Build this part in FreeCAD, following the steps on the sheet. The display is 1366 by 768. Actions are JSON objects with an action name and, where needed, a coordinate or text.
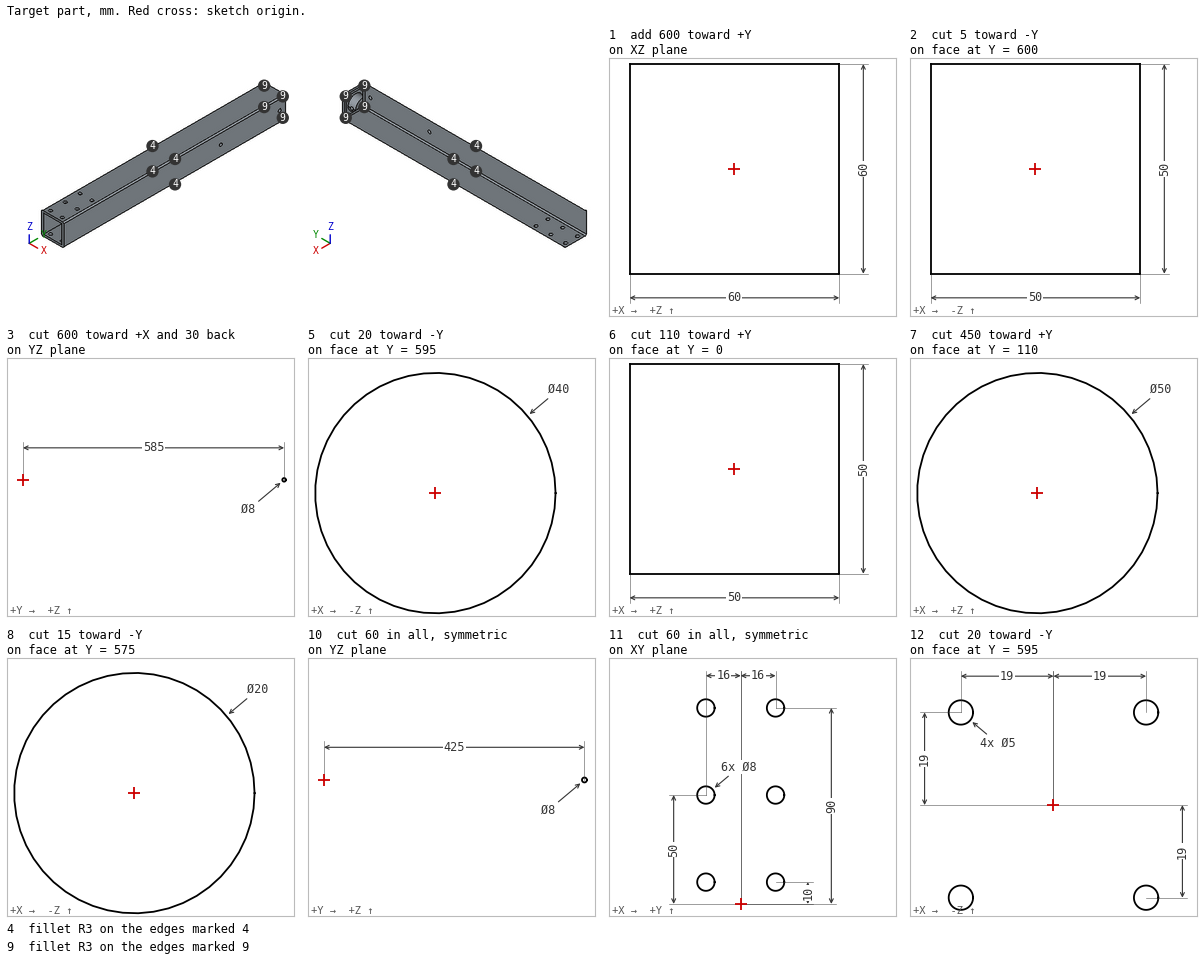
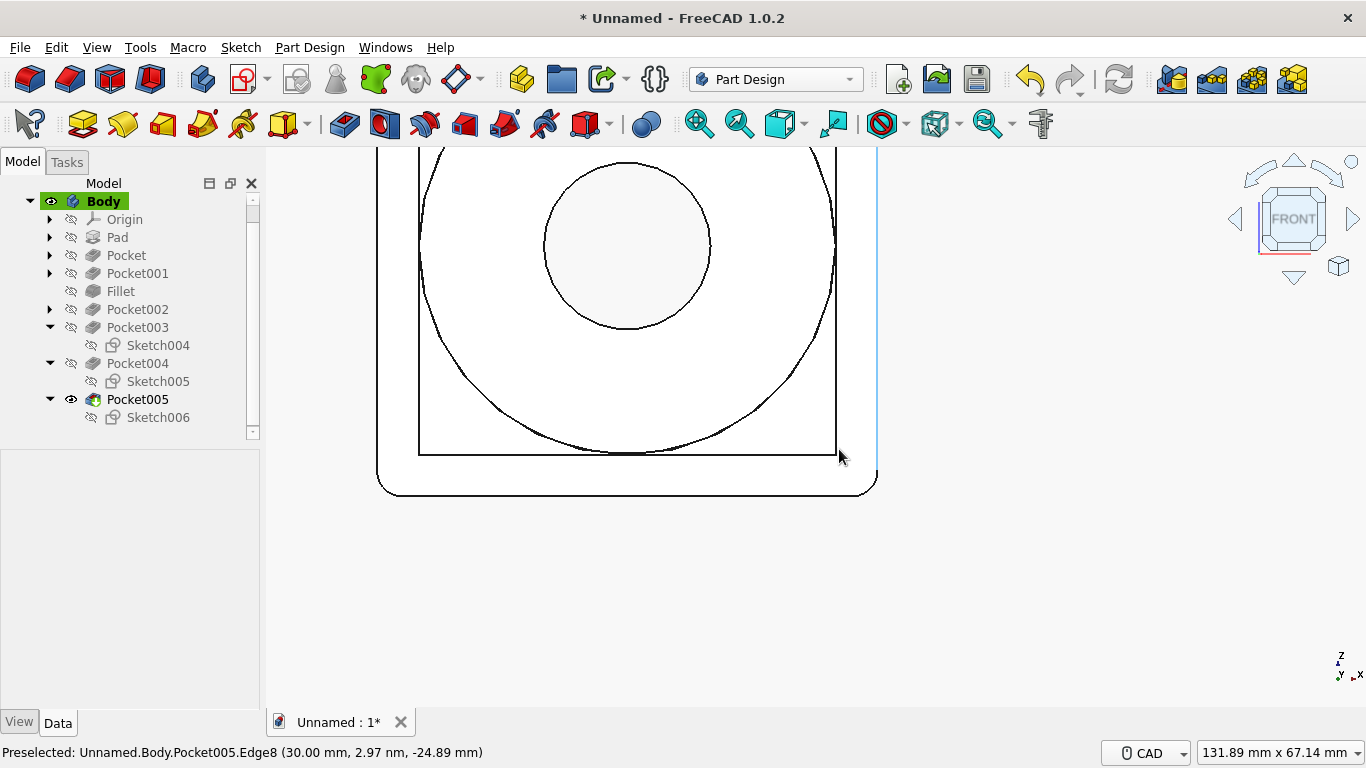
{"action": "left_click", "coordinate": [700, 124]}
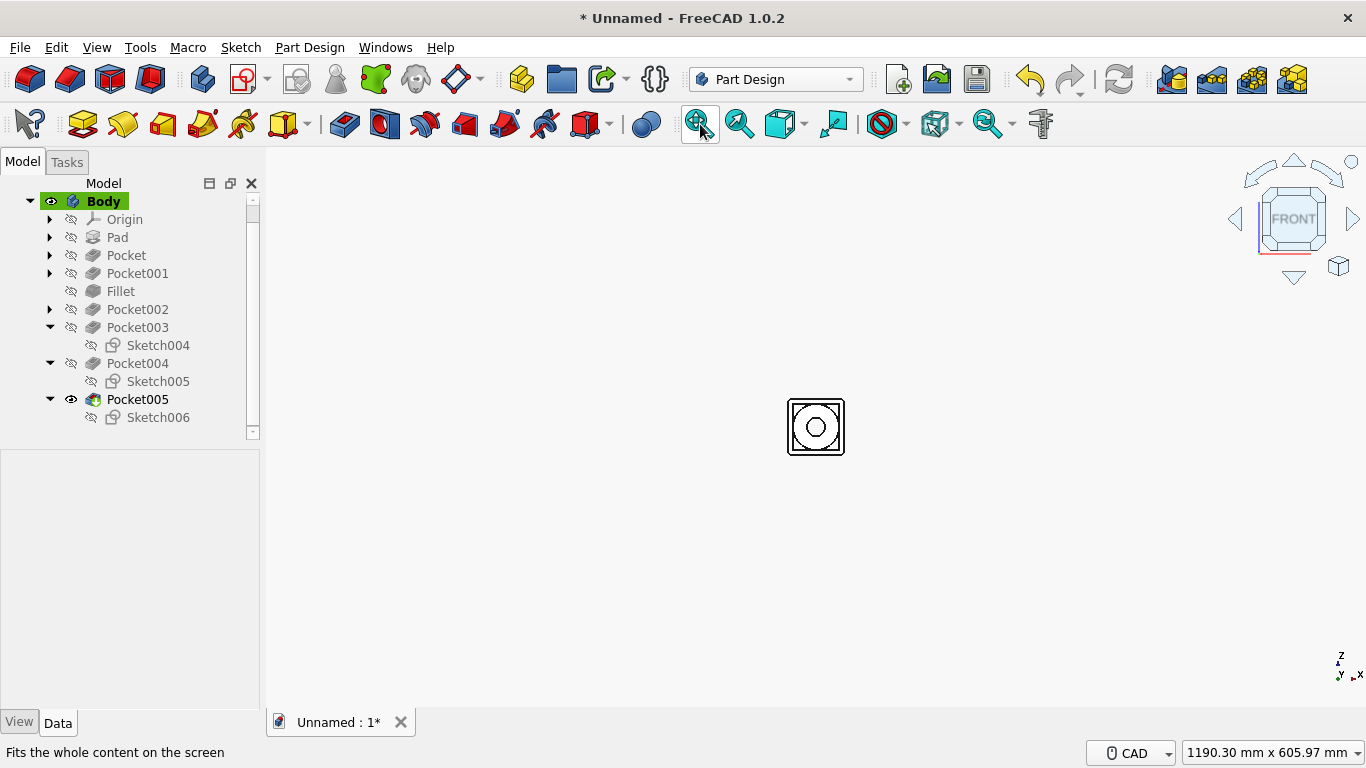
{"action": "key", "text": "3"}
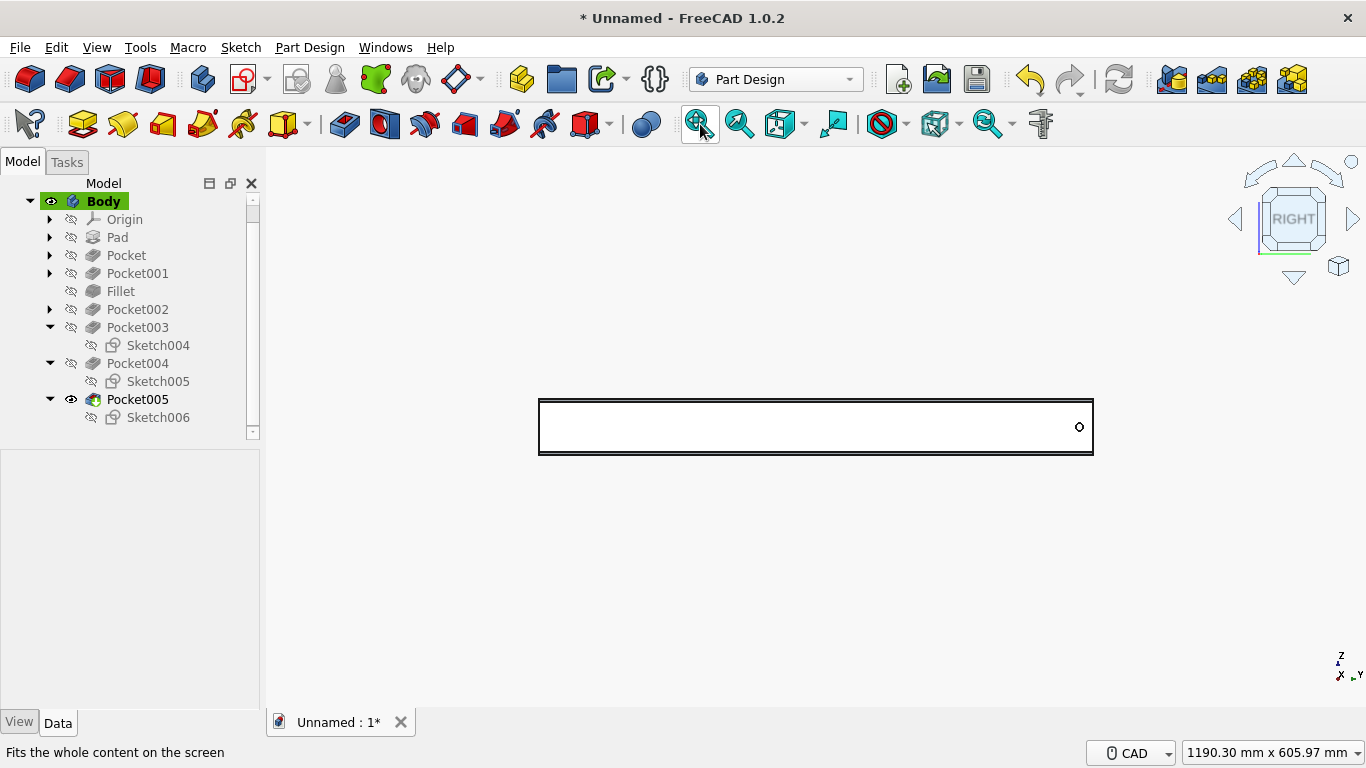
{"action": "scroll", "coordinate": [1091, 449], "scroll_direction": "up", "scroll_amount": 11}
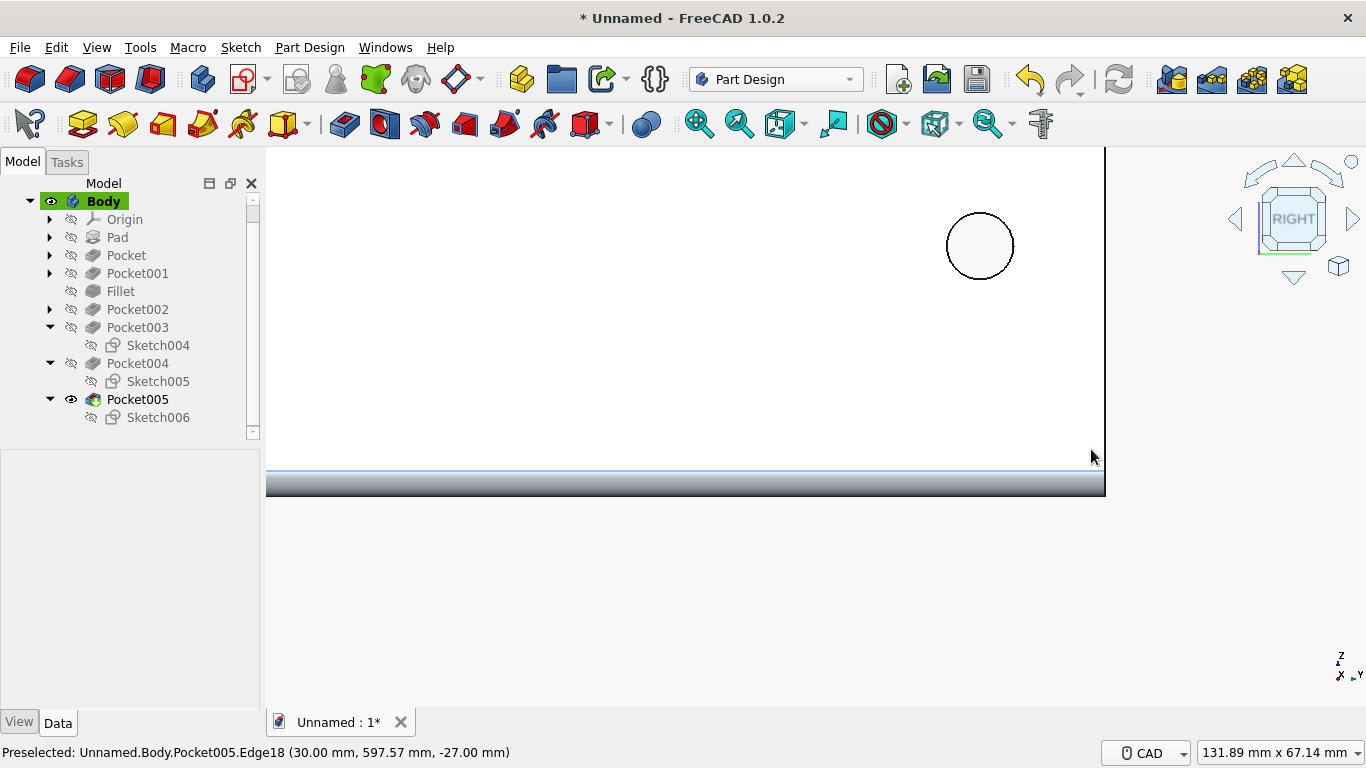
{"action": "left_click", "coordinate": [700, 124]}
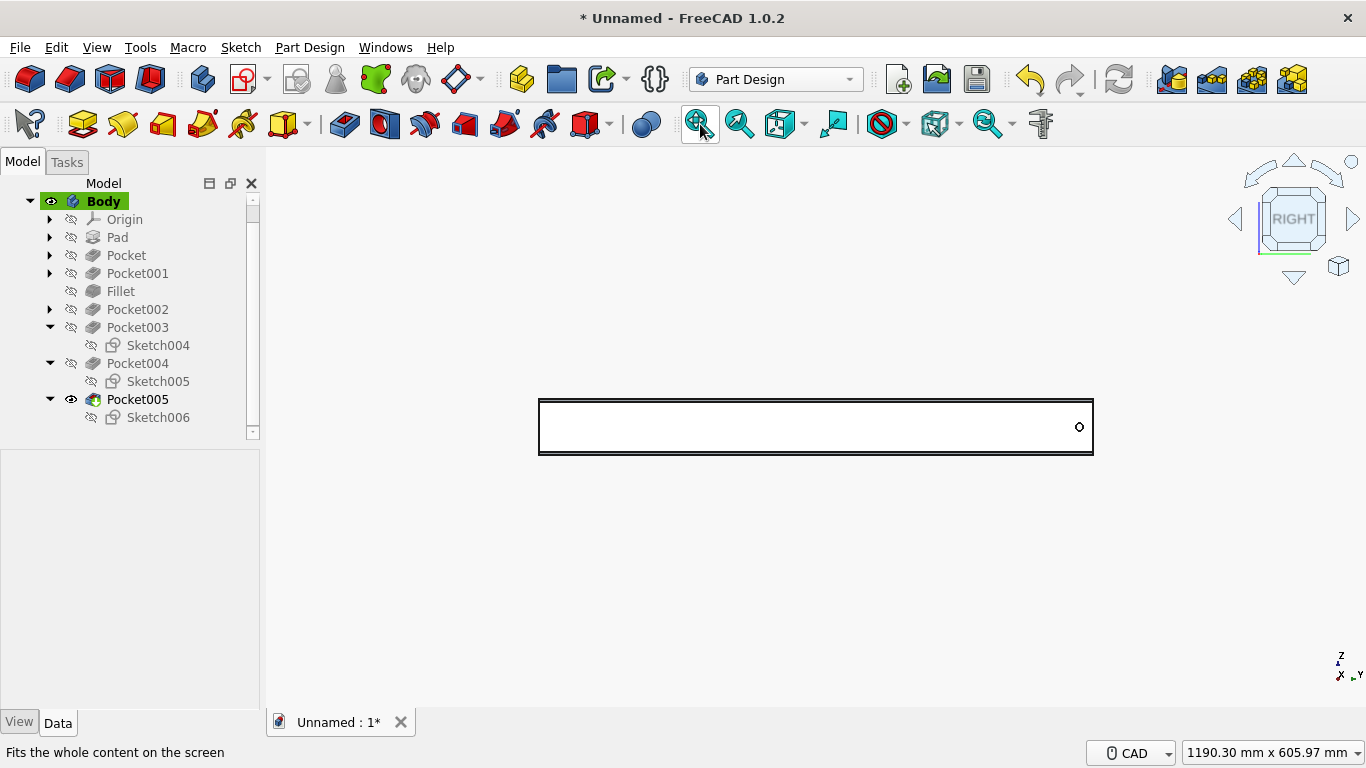
{"action": "key", "text": "5"}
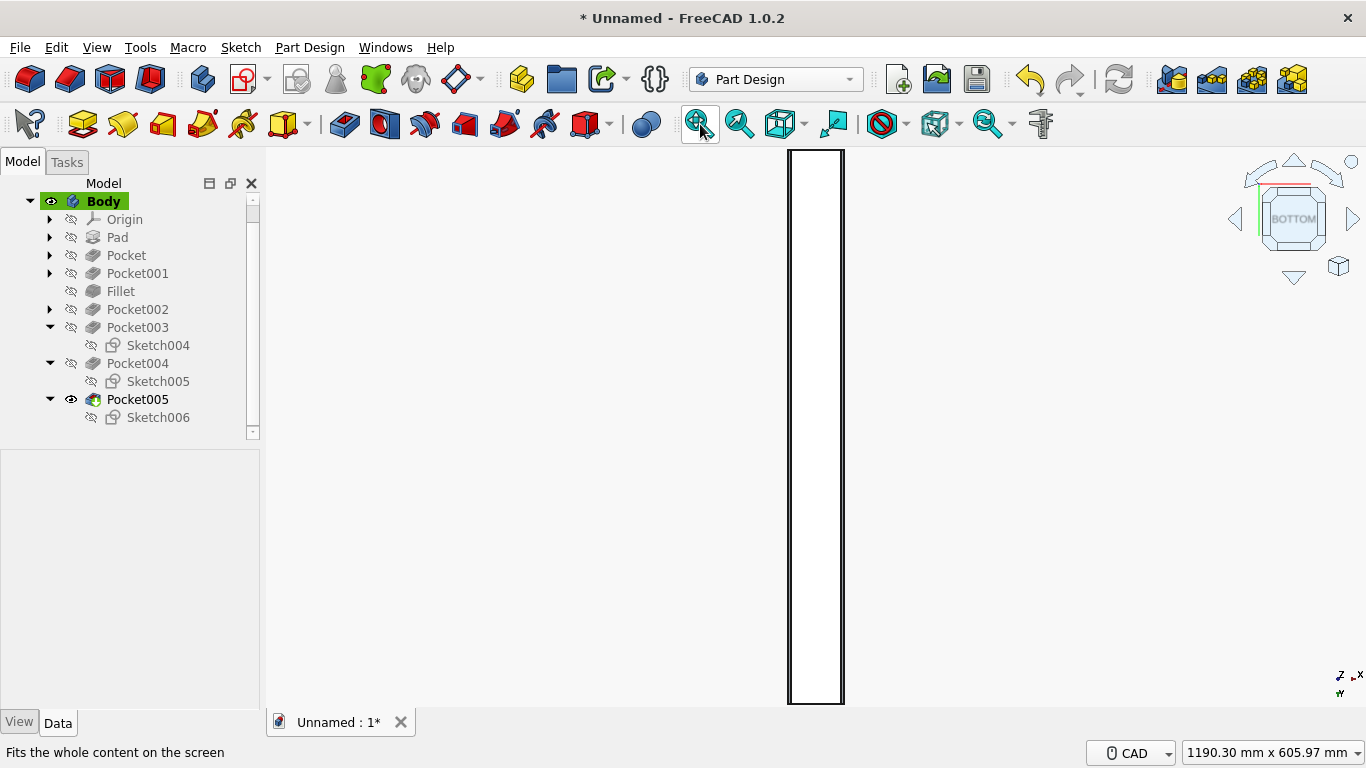
{"action": "key", "text": "4"}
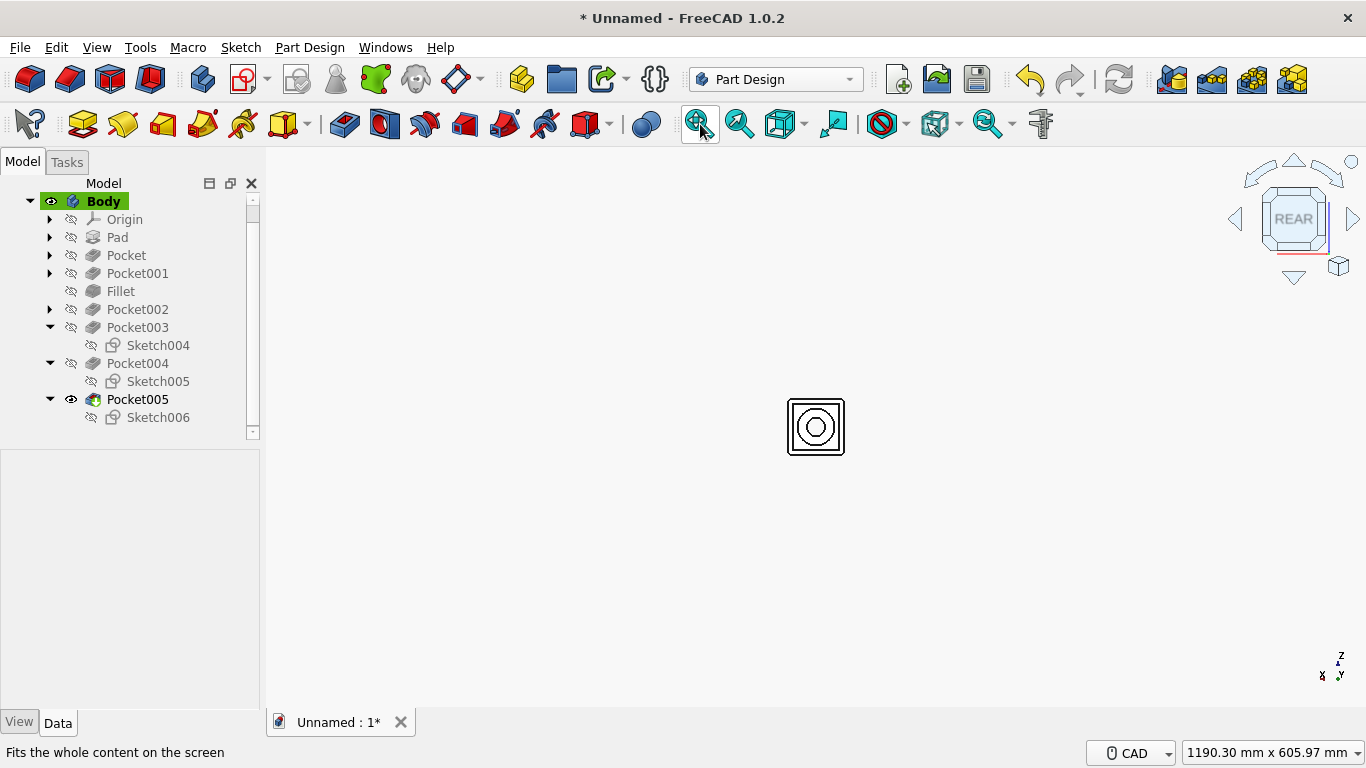
{"action": "left_click", "coordinate": [700, 124]}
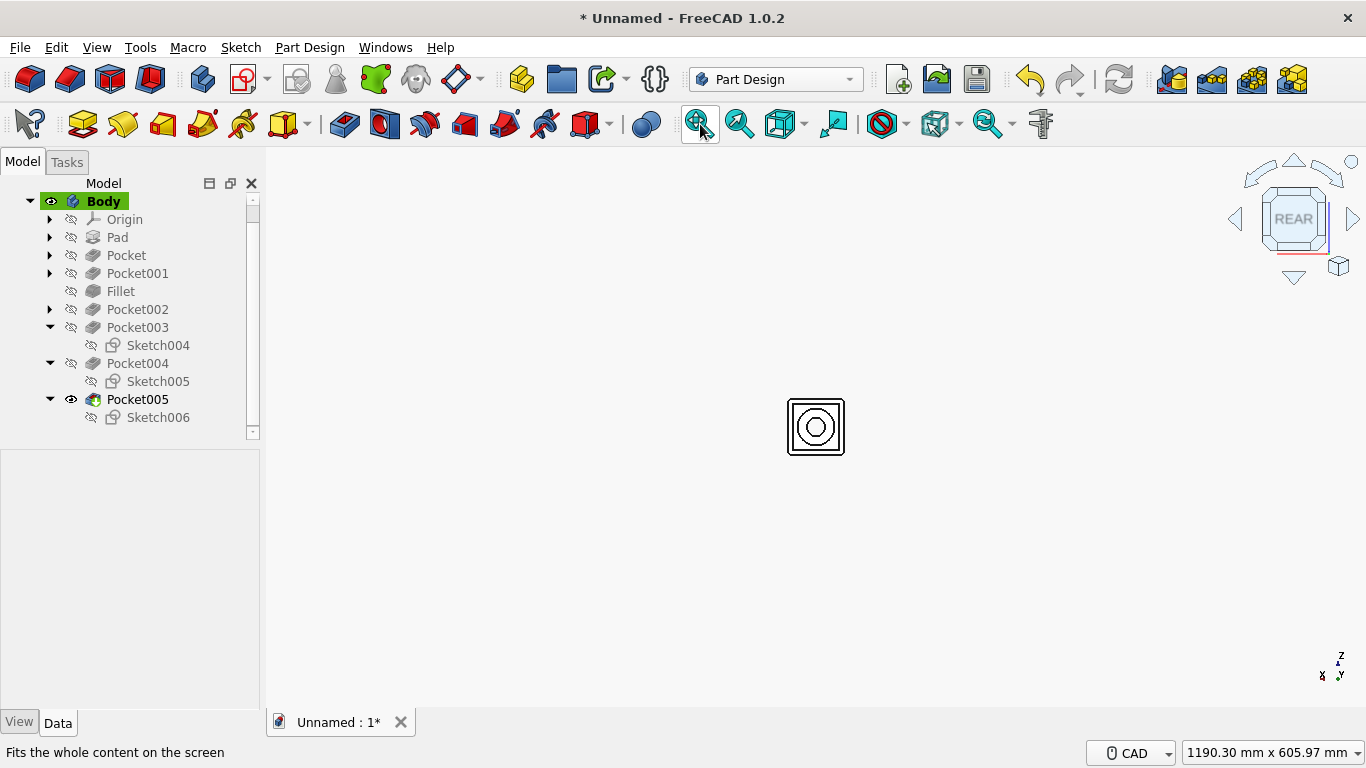
{"action": "scroll", "coordinate": [793, 449], "scroll_direction": "up", "scroll_amount": 11}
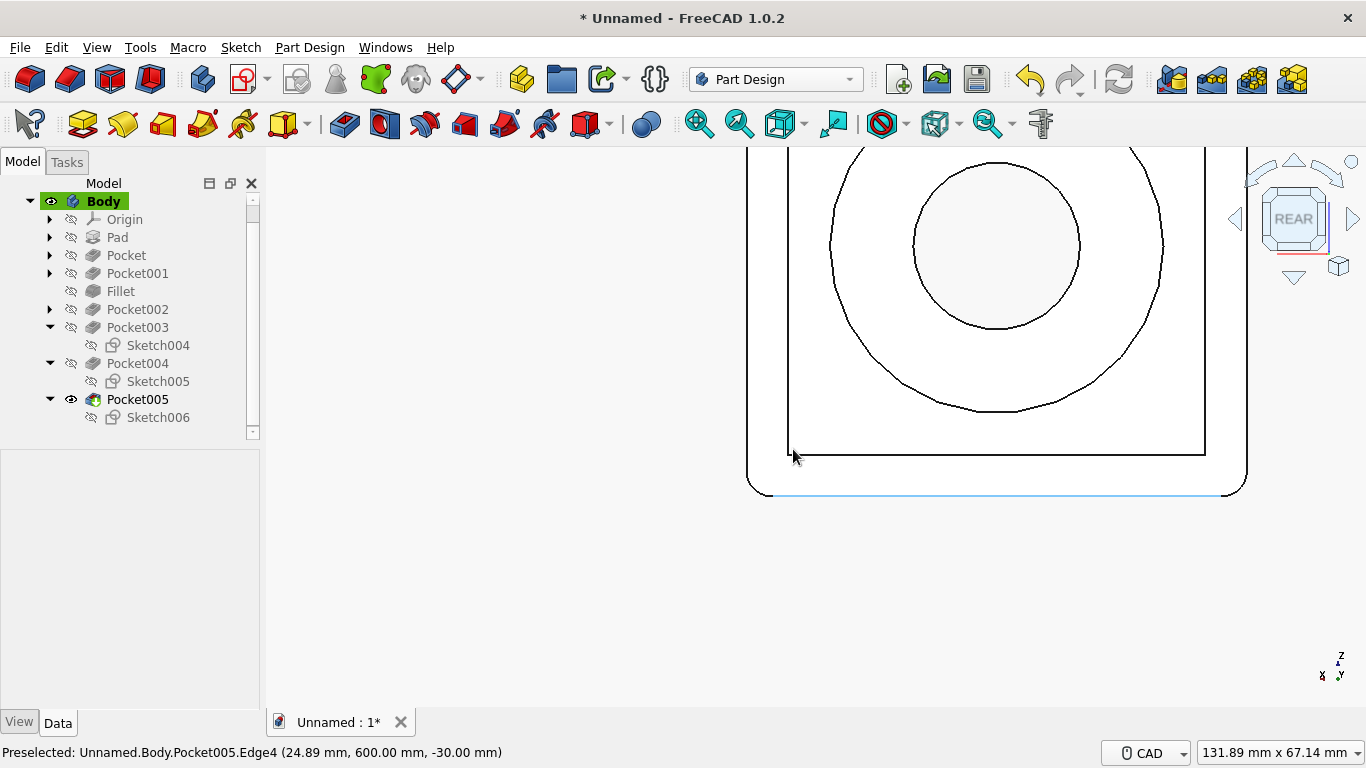
{"action": "left_click", "coordinate": [700, 124]}